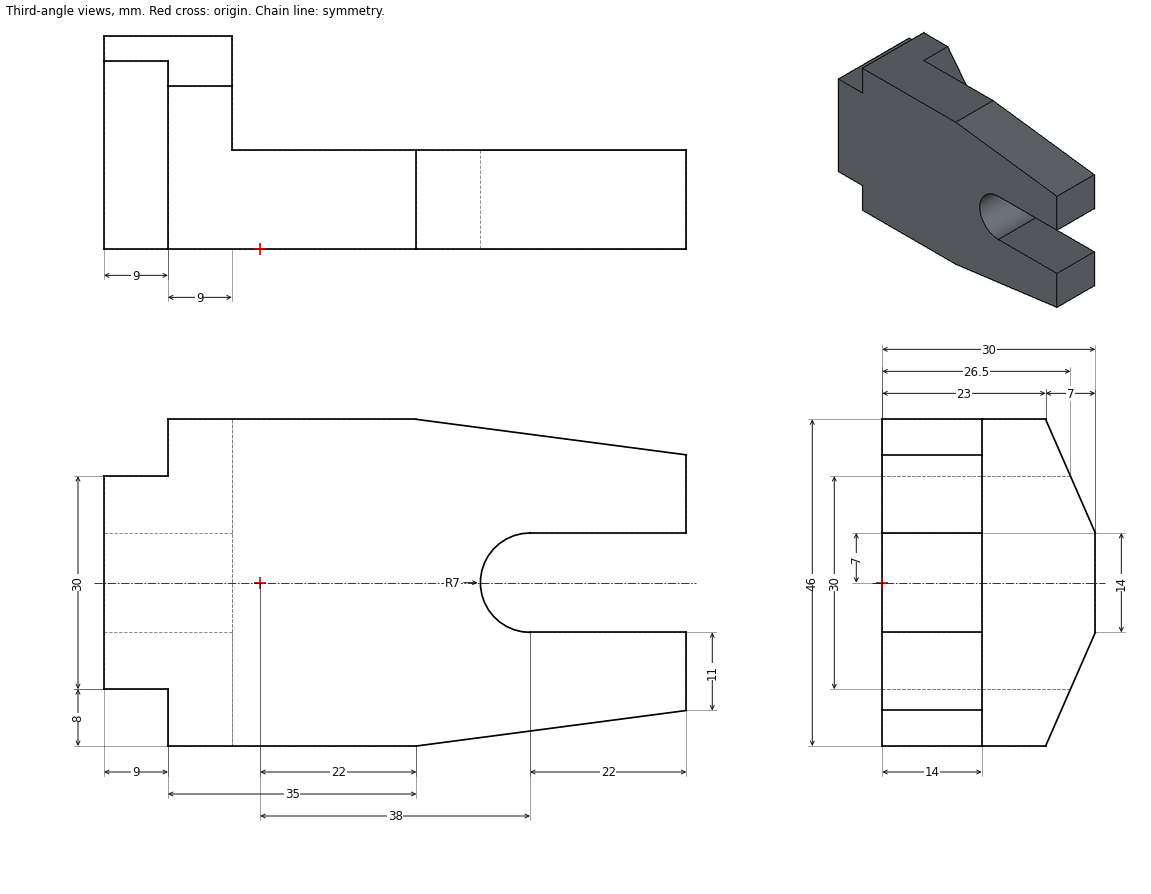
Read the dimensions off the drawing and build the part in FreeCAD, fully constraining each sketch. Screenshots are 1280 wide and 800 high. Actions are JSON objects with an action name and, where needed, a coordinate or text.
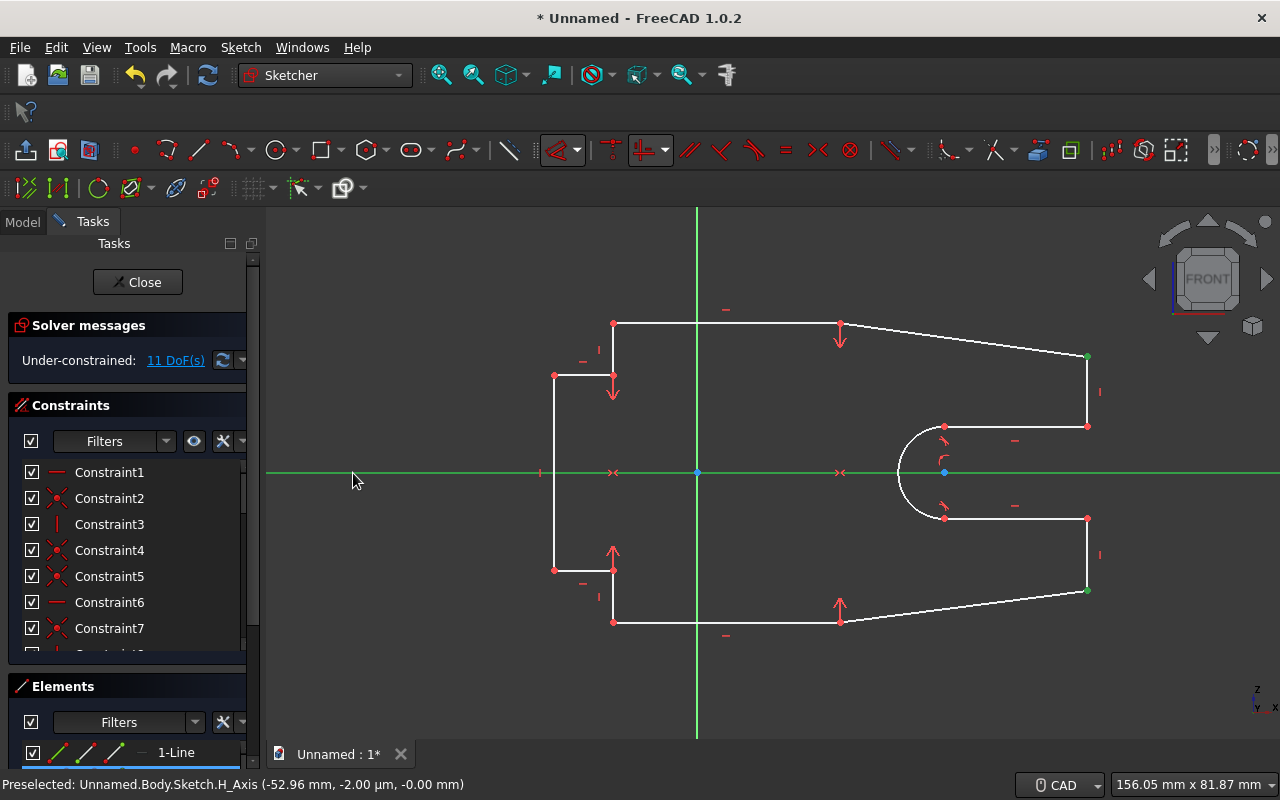
{"action": "left_click", "coordinate": [818, 150]}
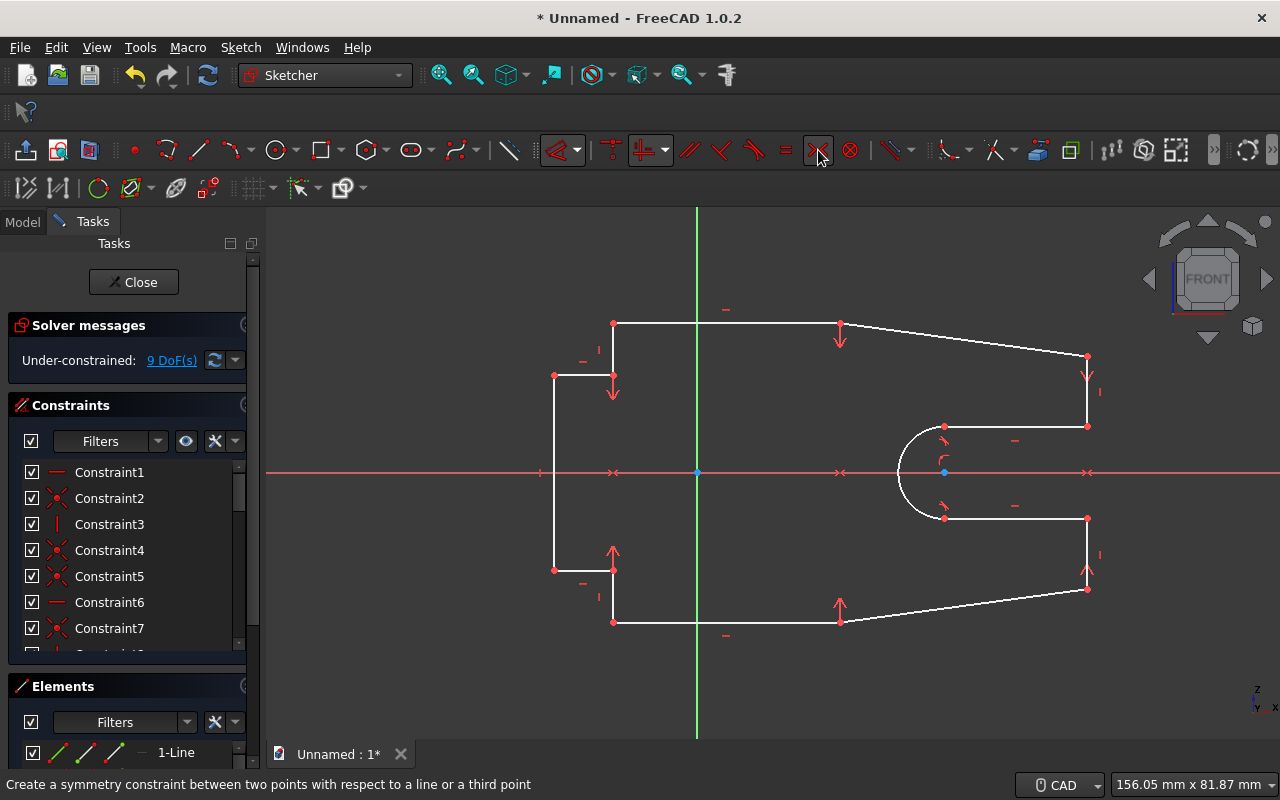
{"action": "key", "text": "d"}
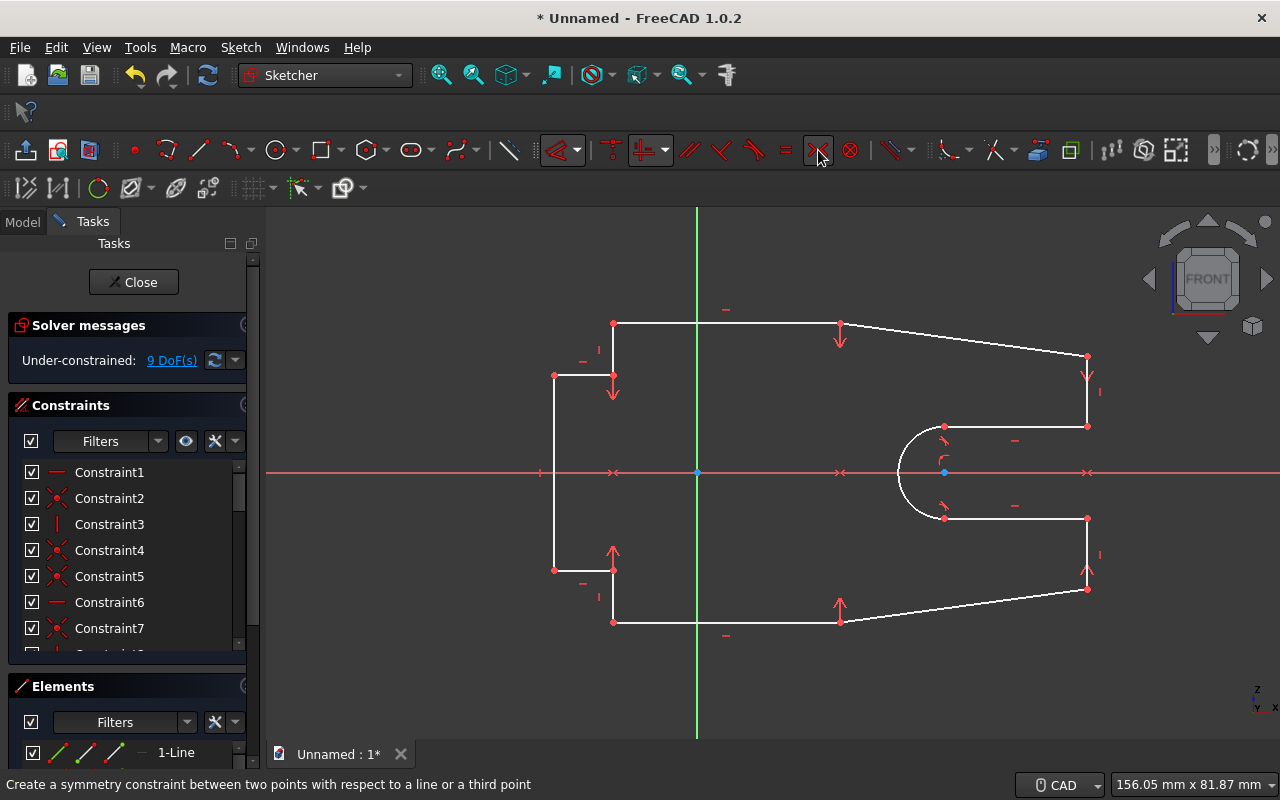
{"action": "left_click", "coordinate": [907, 446]}
{"action": "left_click", "coordinate": [881, 427]}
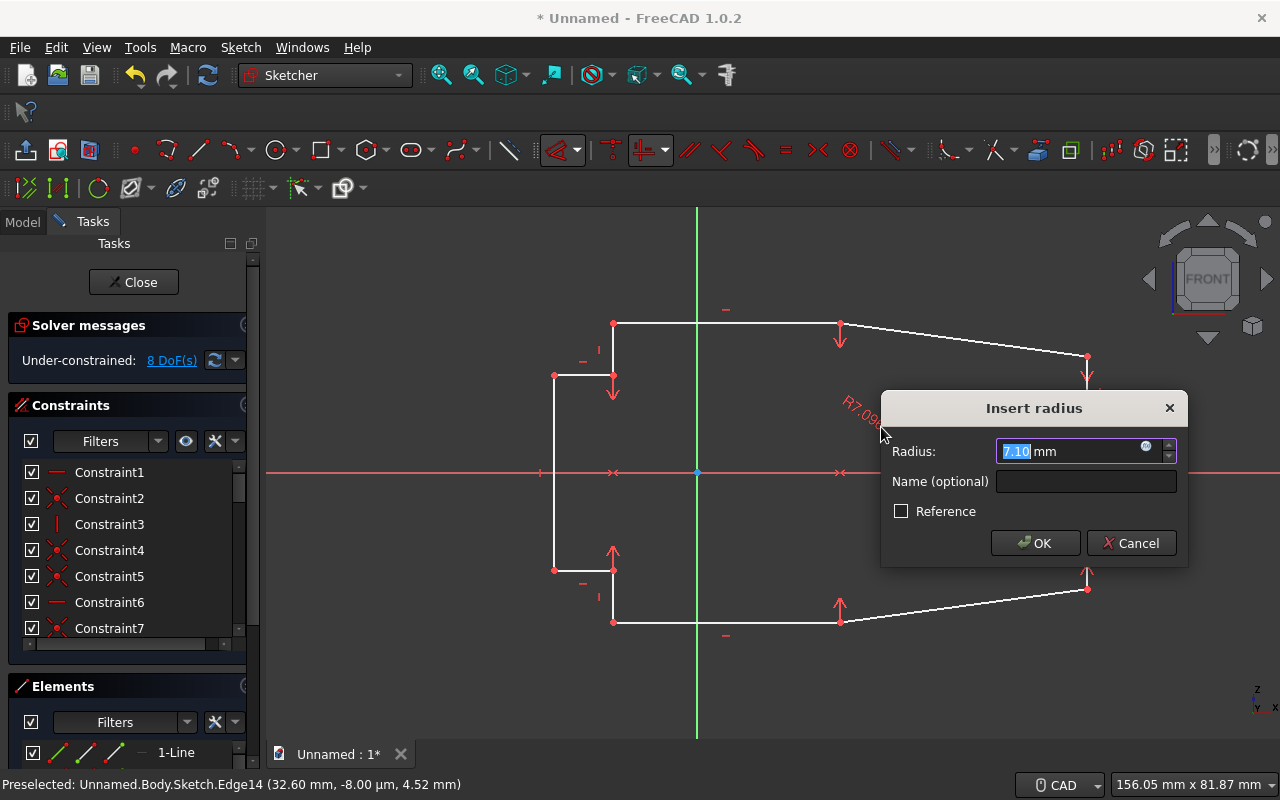
{"action": "type", "text": "7"}
{"action": "key", "text": "Return"}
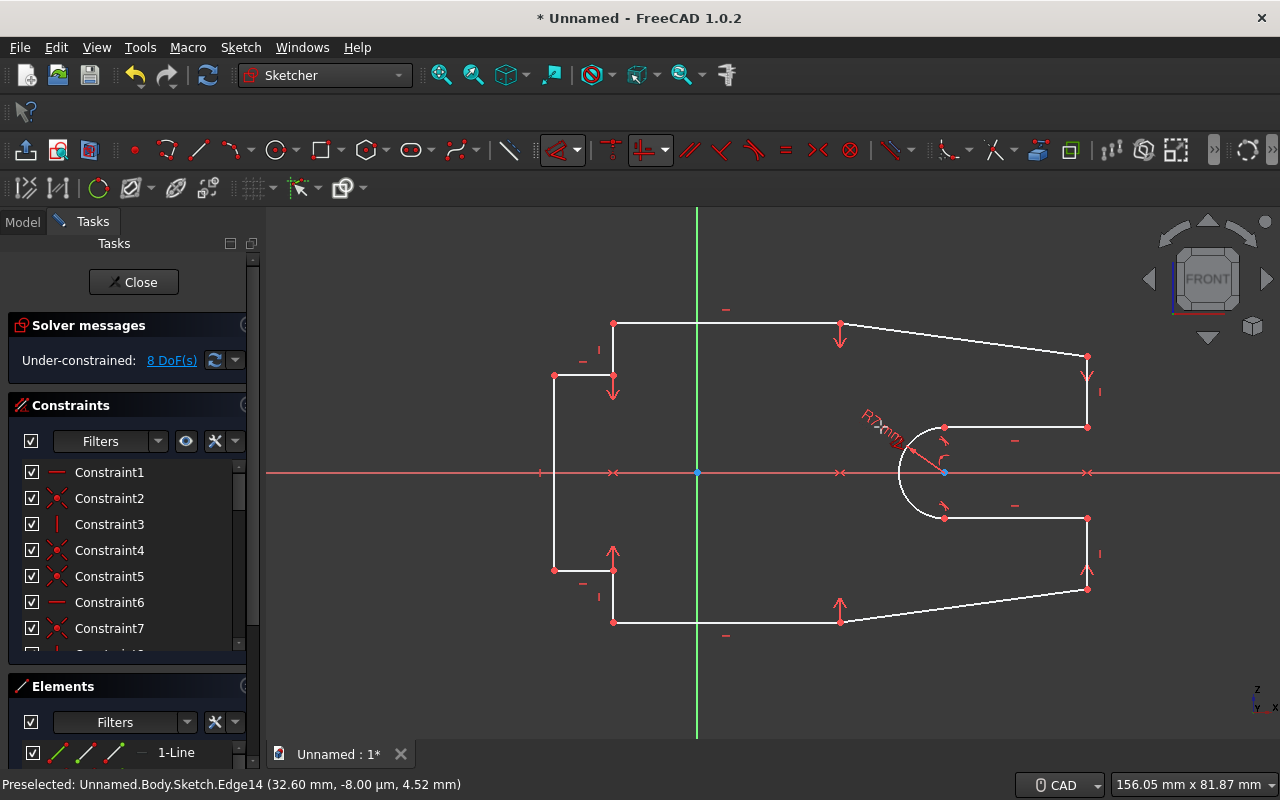
{"action": "left_click", "coordinate": [613, 607]}
{"action": "left_click", "coordinate": [579, 597]}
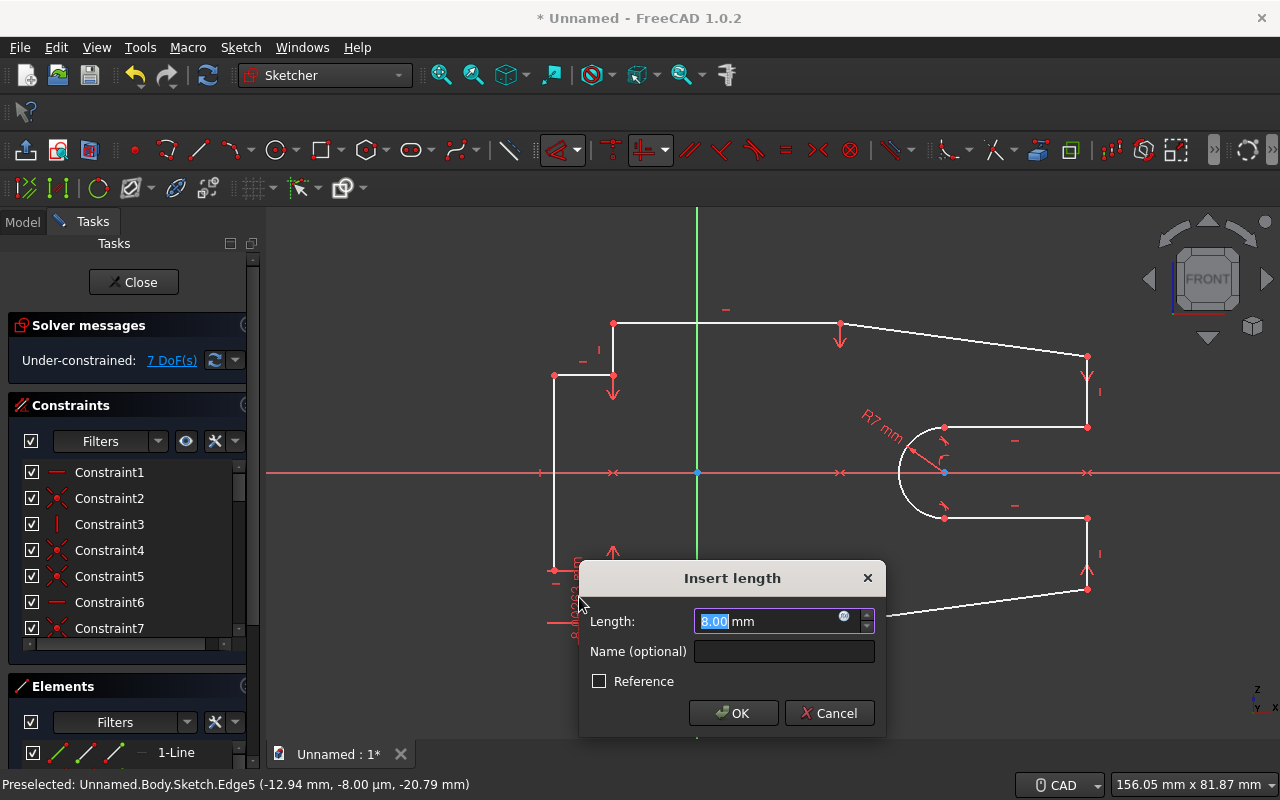
{"action": "type", "text": "8"}
{"action": "key", "text": "Return"}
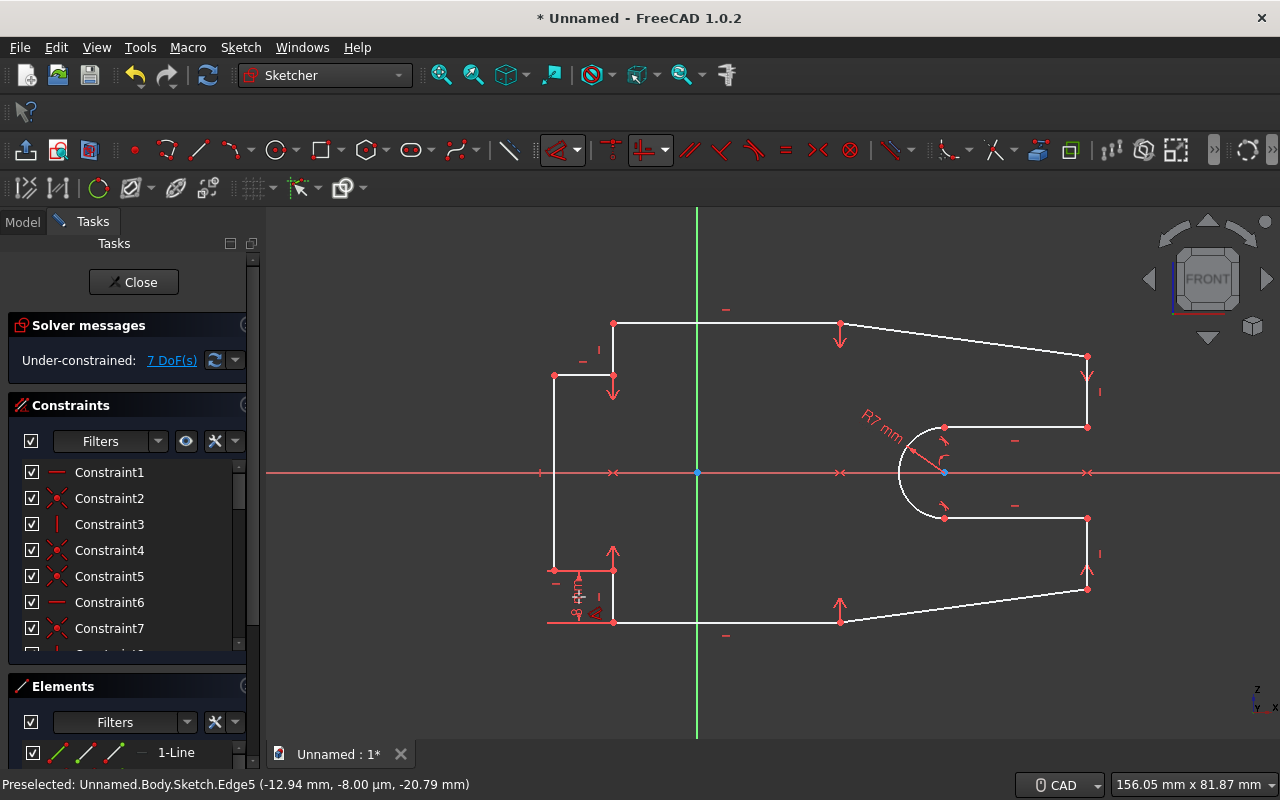
{"action": "left_click", "coordinate": [595, 571]}
{"action": "left_click", "coordinate": [583, 537]}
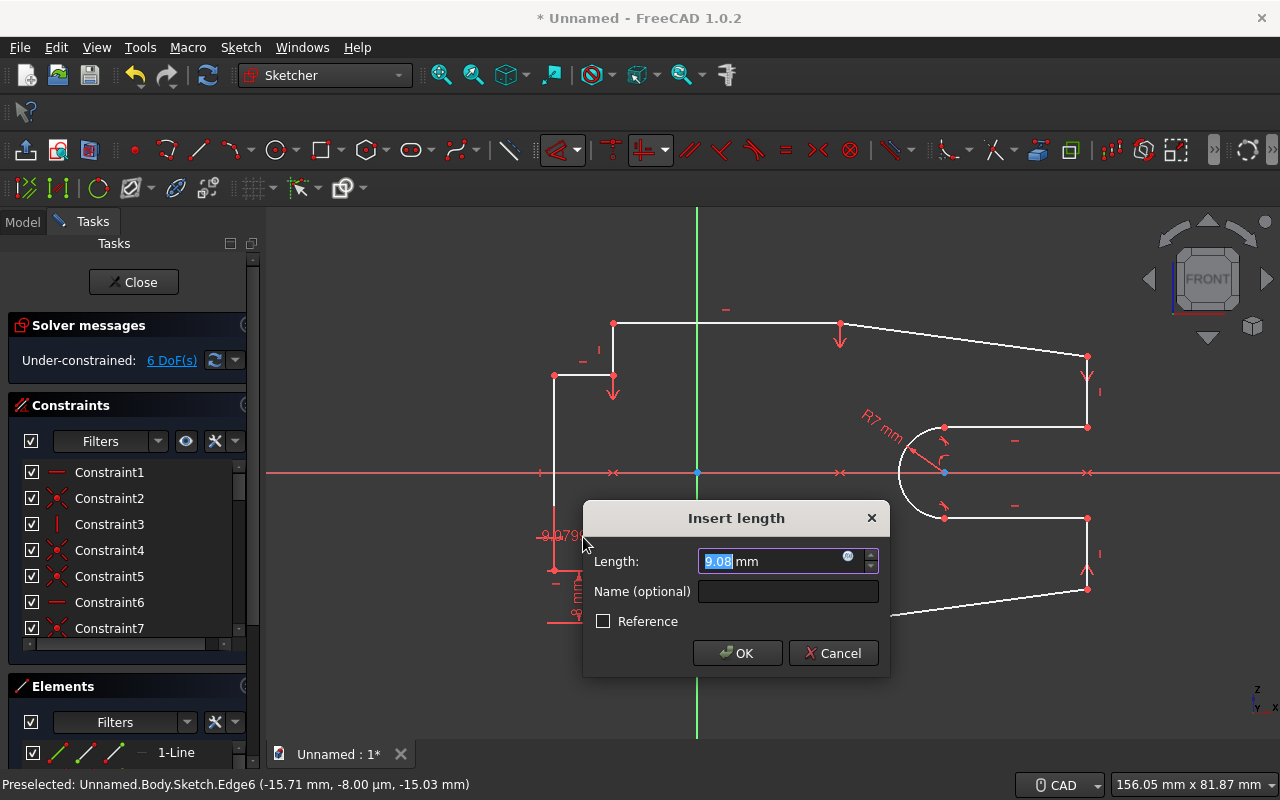
{"action": "type", "text": "9"}
{"action": "key", "text": "Return"}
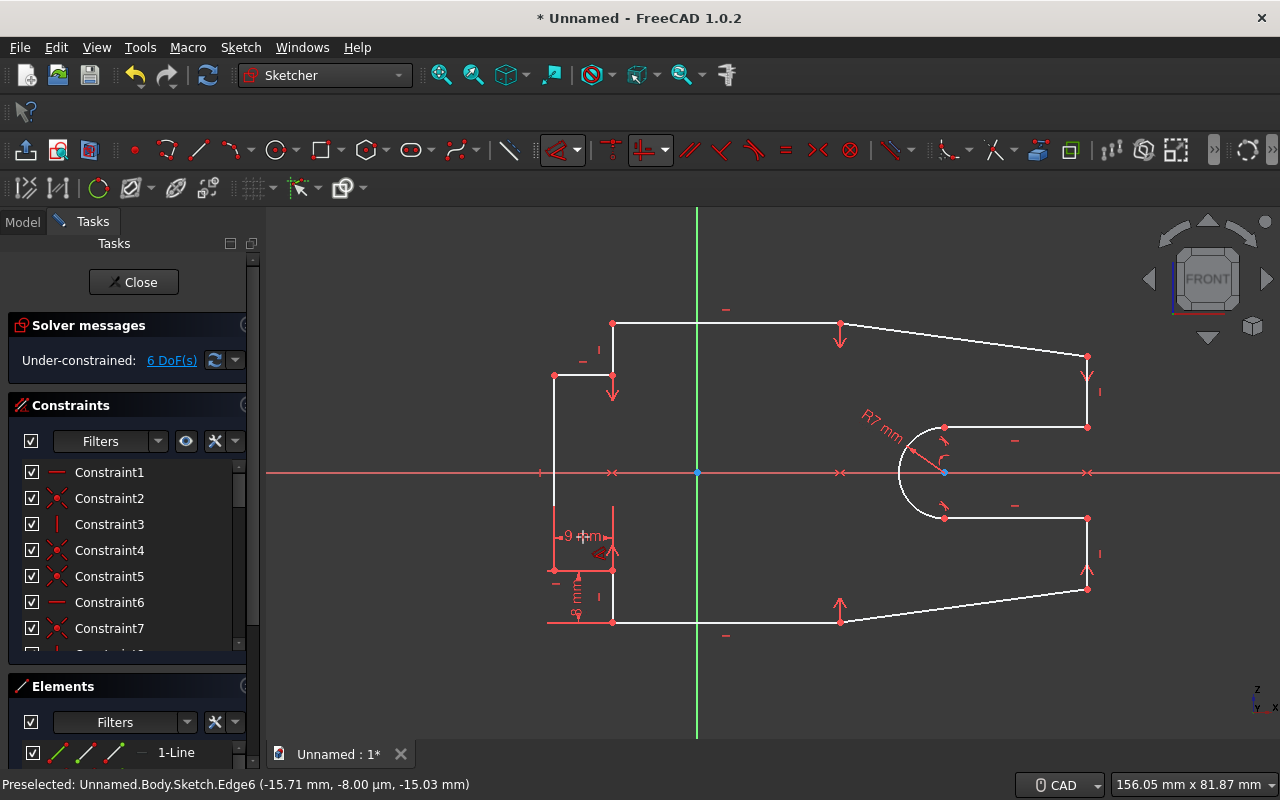
{"action": "left_click", "coordinate": [987, 518]}
{"action": "left_click", "coordinate": [1016, 552]}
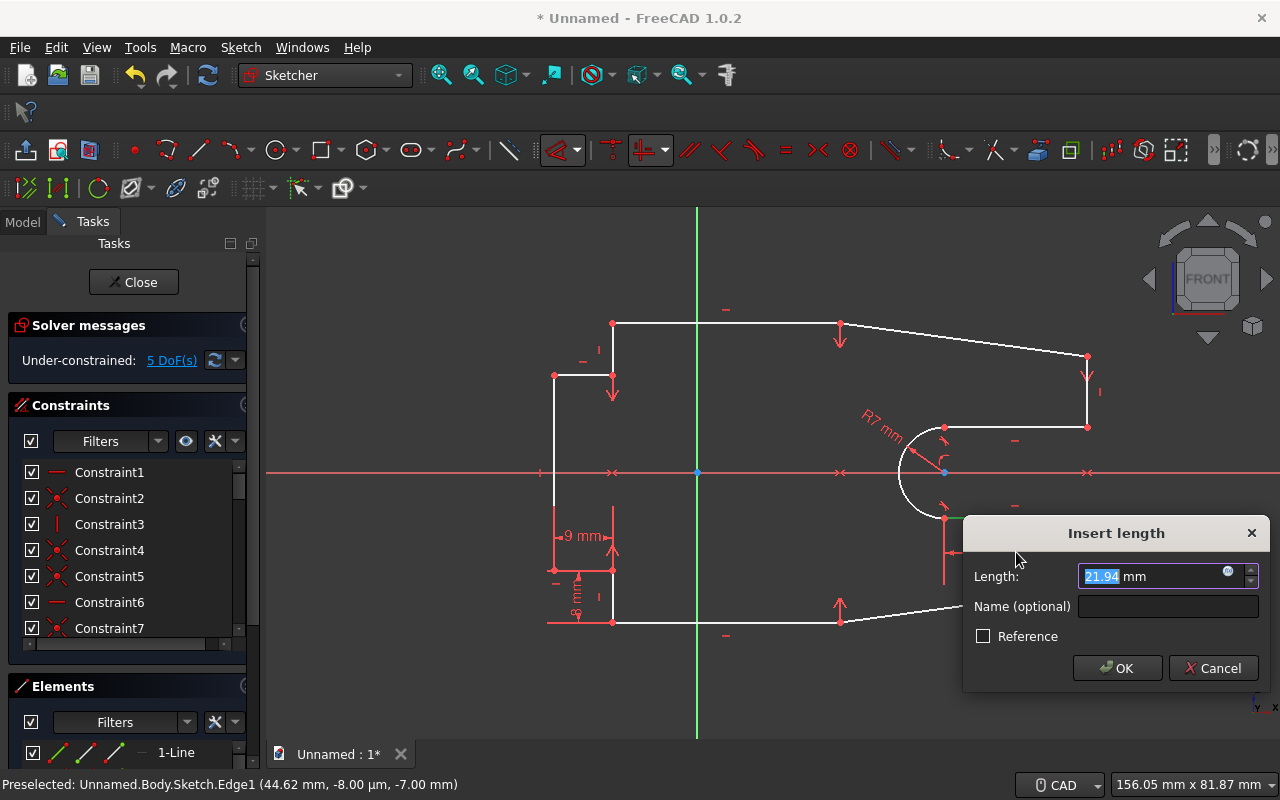
{"action": "type", "text": "22"}
{"action": "key", "text": "Return"}